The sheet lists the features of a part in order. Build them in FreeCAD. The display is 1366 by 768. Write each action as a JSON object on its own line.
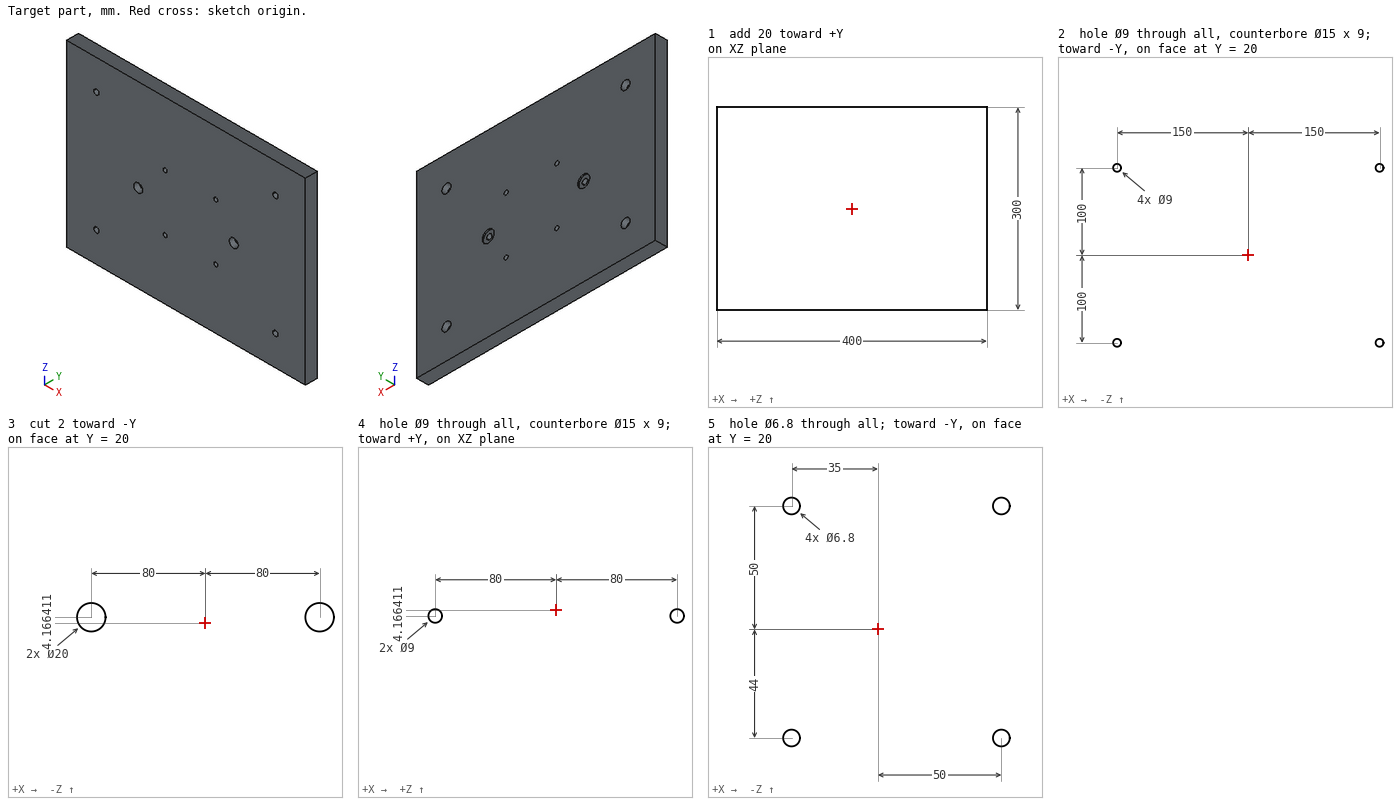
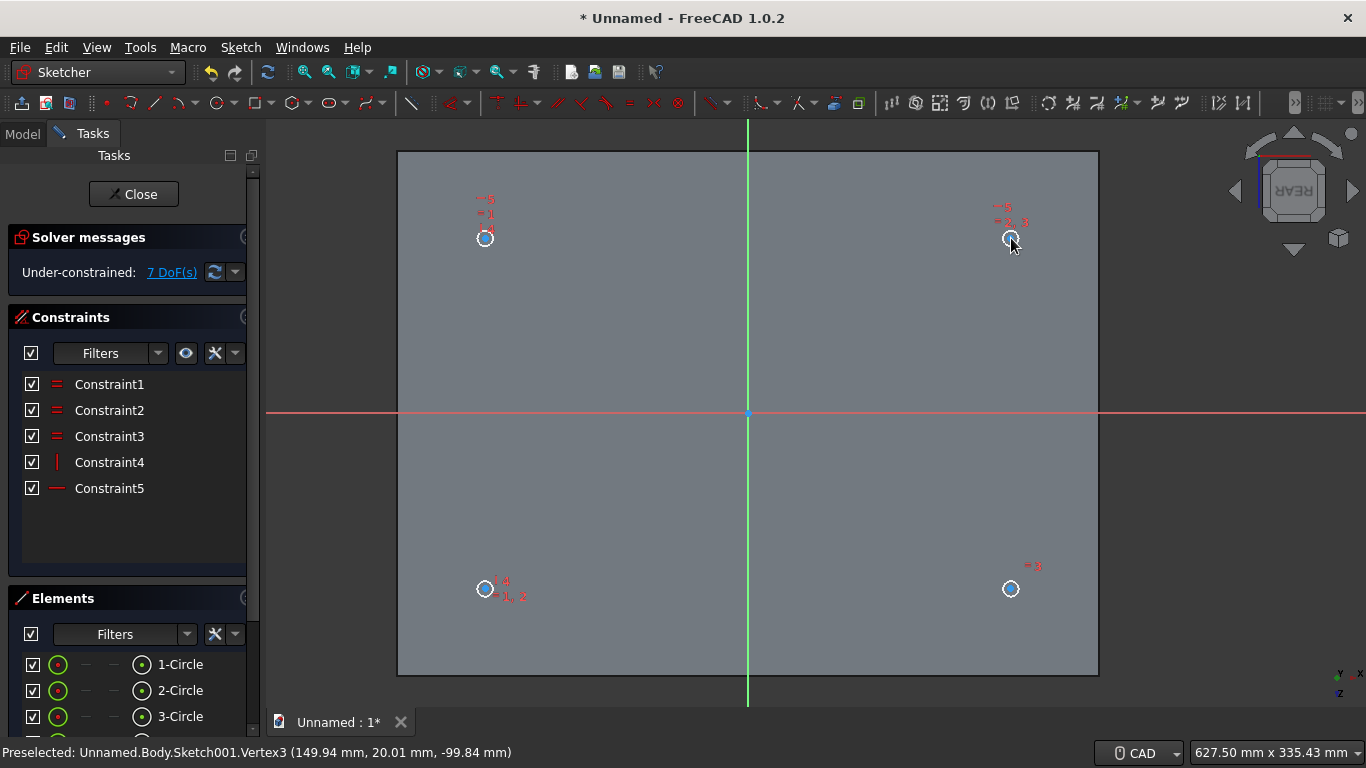
{"action": "left_click", "coordinate": [1011, 238]}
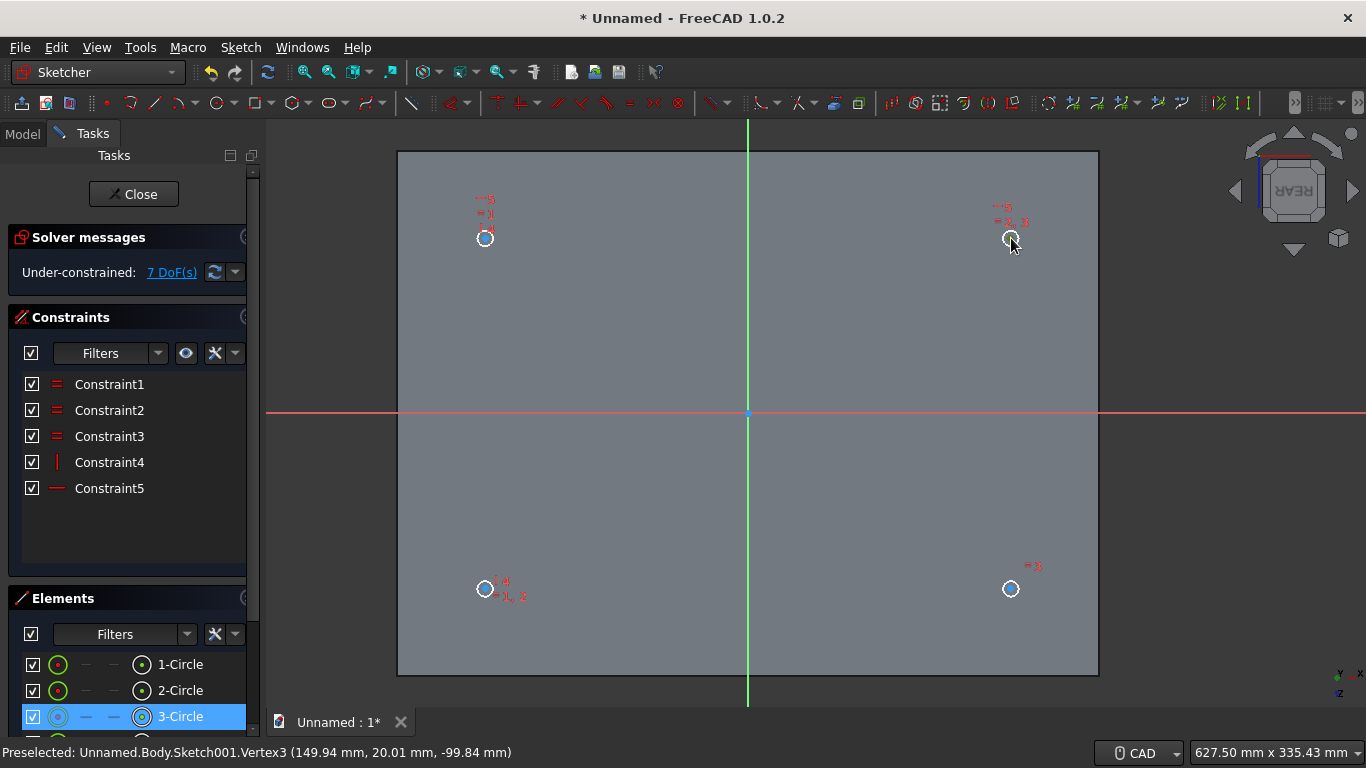
{"action": "left_click", "coordinate": [1011, 589]}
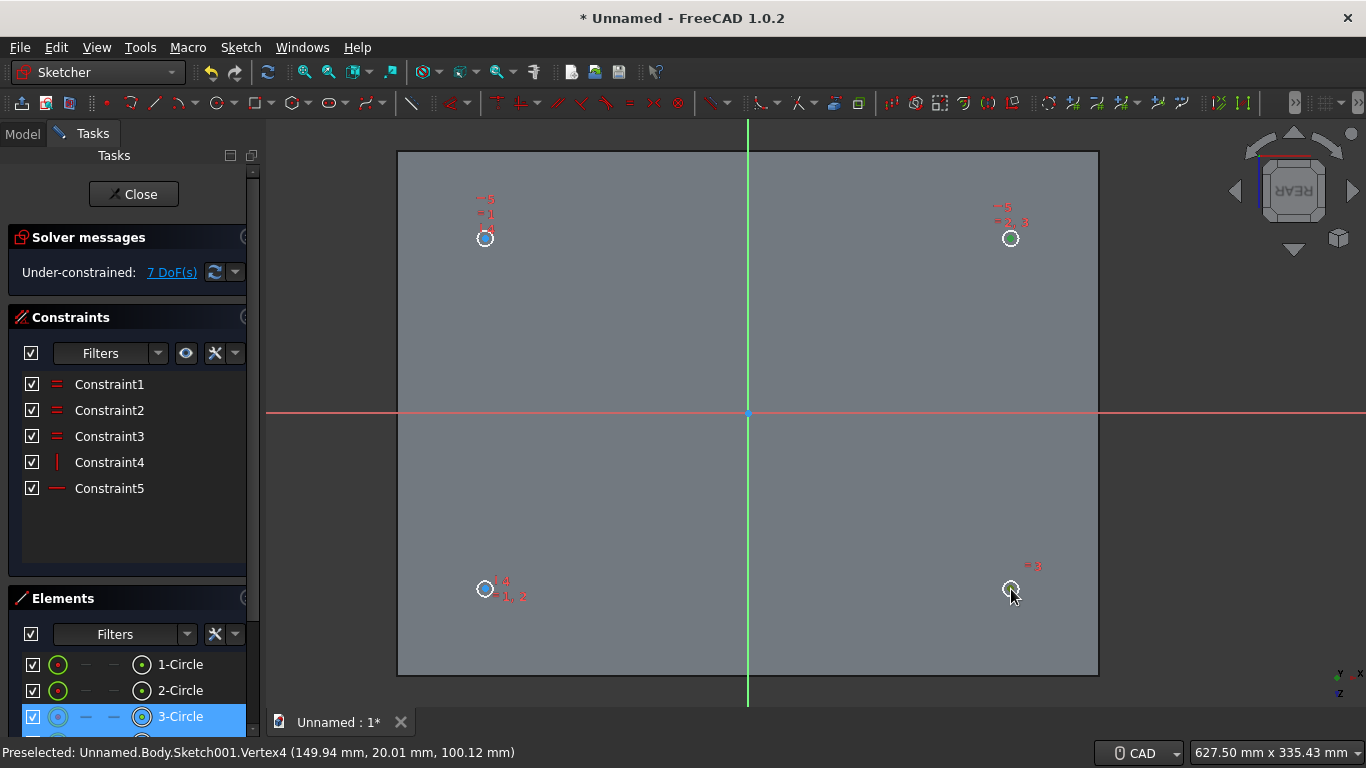
{"action": "key", "text": "v"}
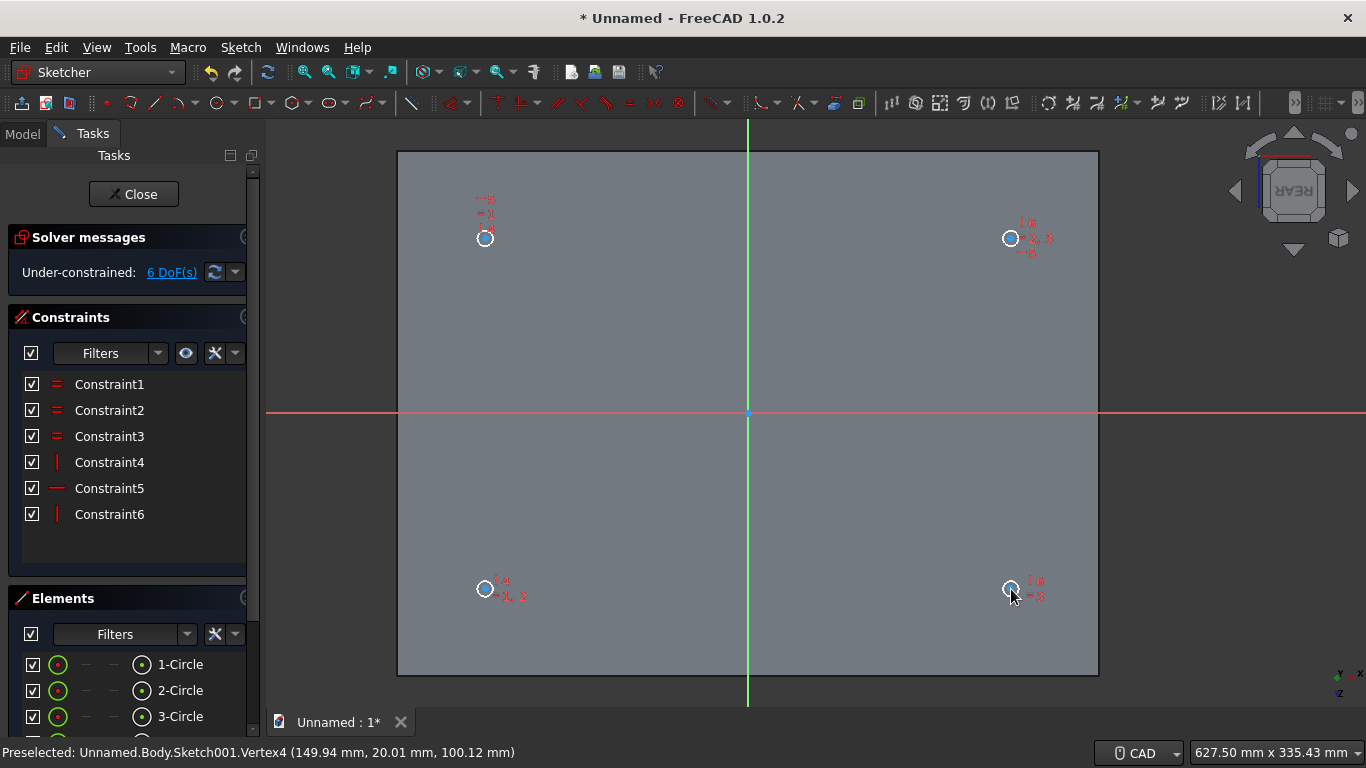
{"action": "left_click", "coordinate": [485, 589]}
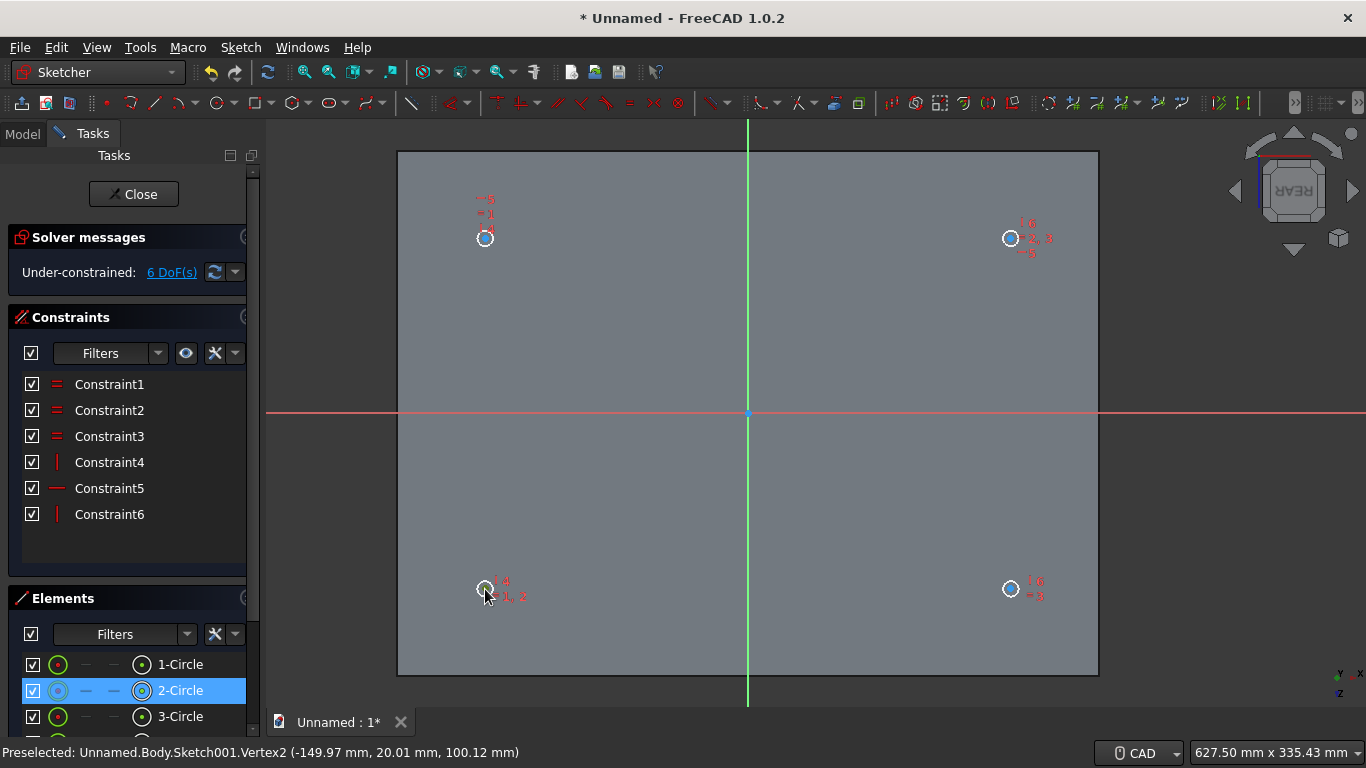
{"action": "left_click", "coordinate": [1011, 589]}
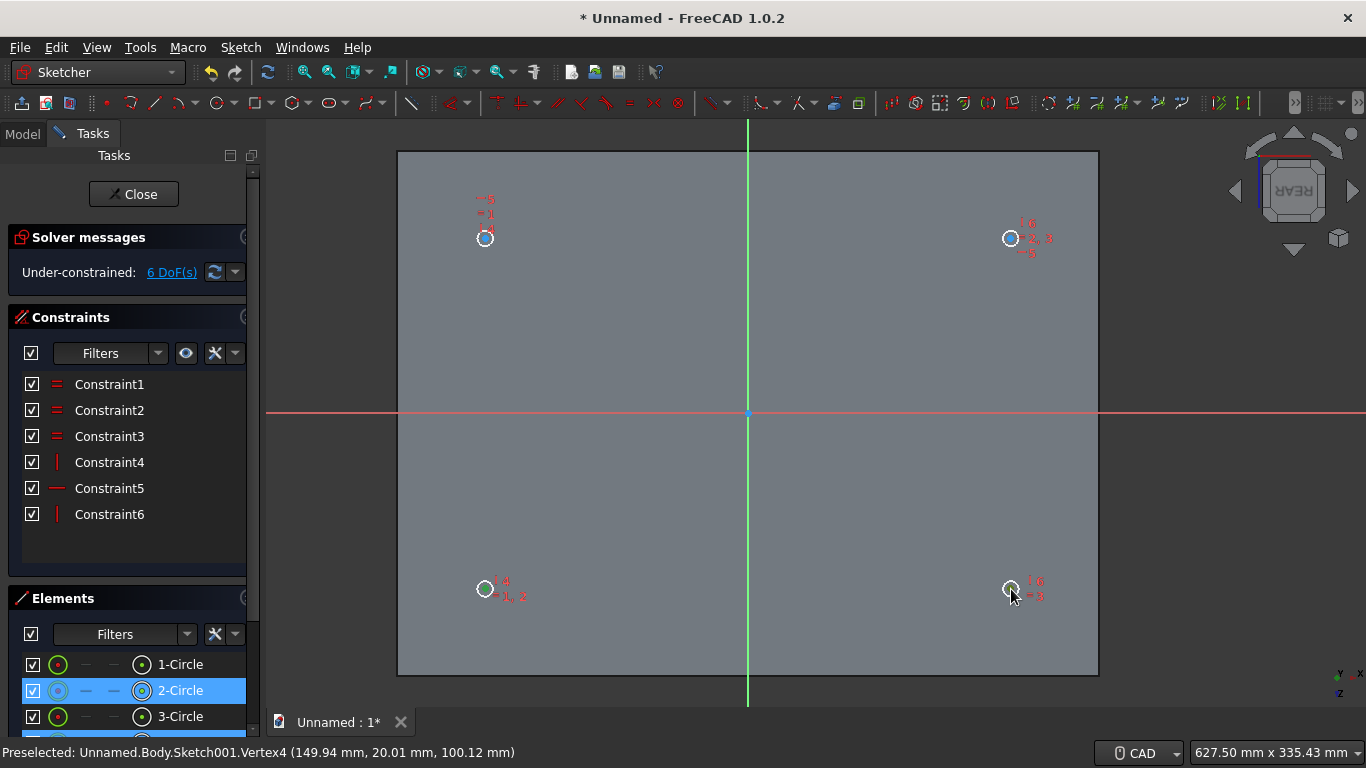
{"action": "left_click", "coordinate": [540, 104]}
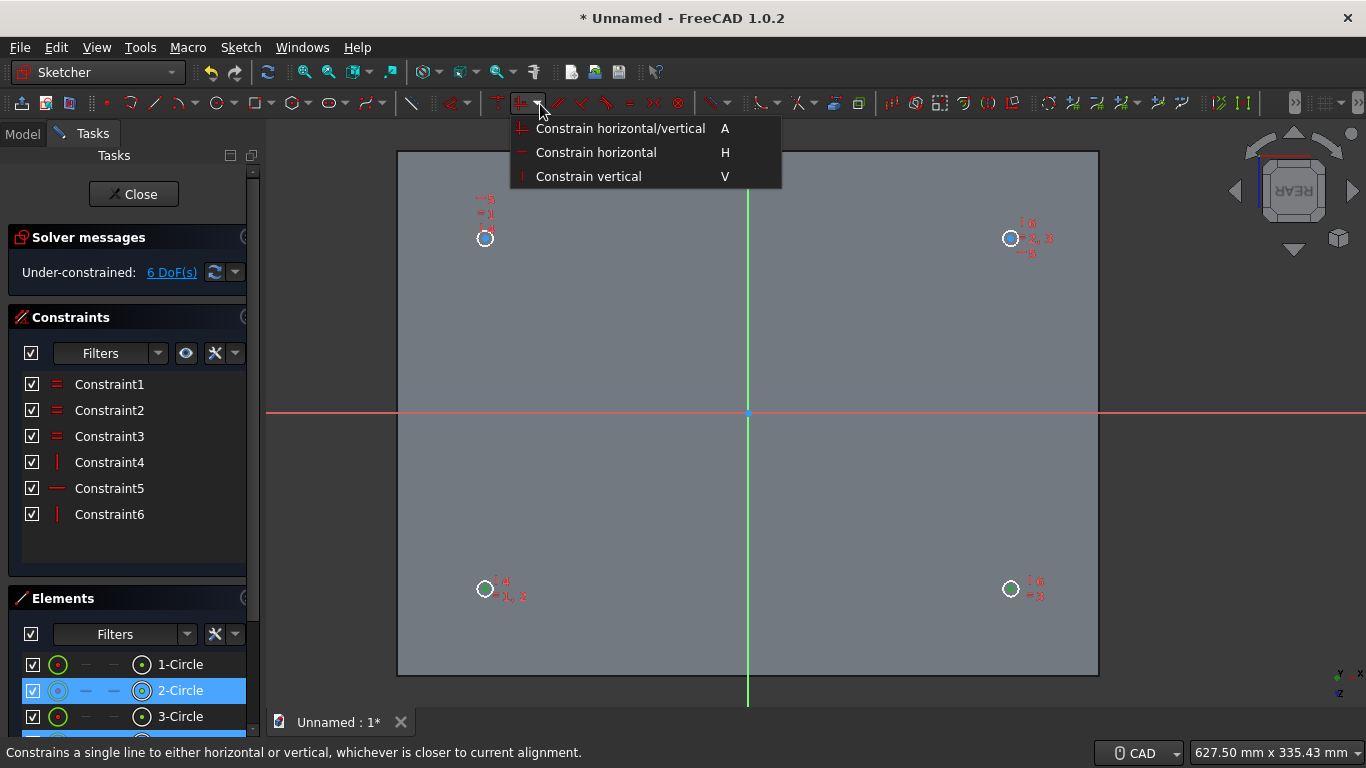
{"action": "left_click", "coordinate": [646, 152]}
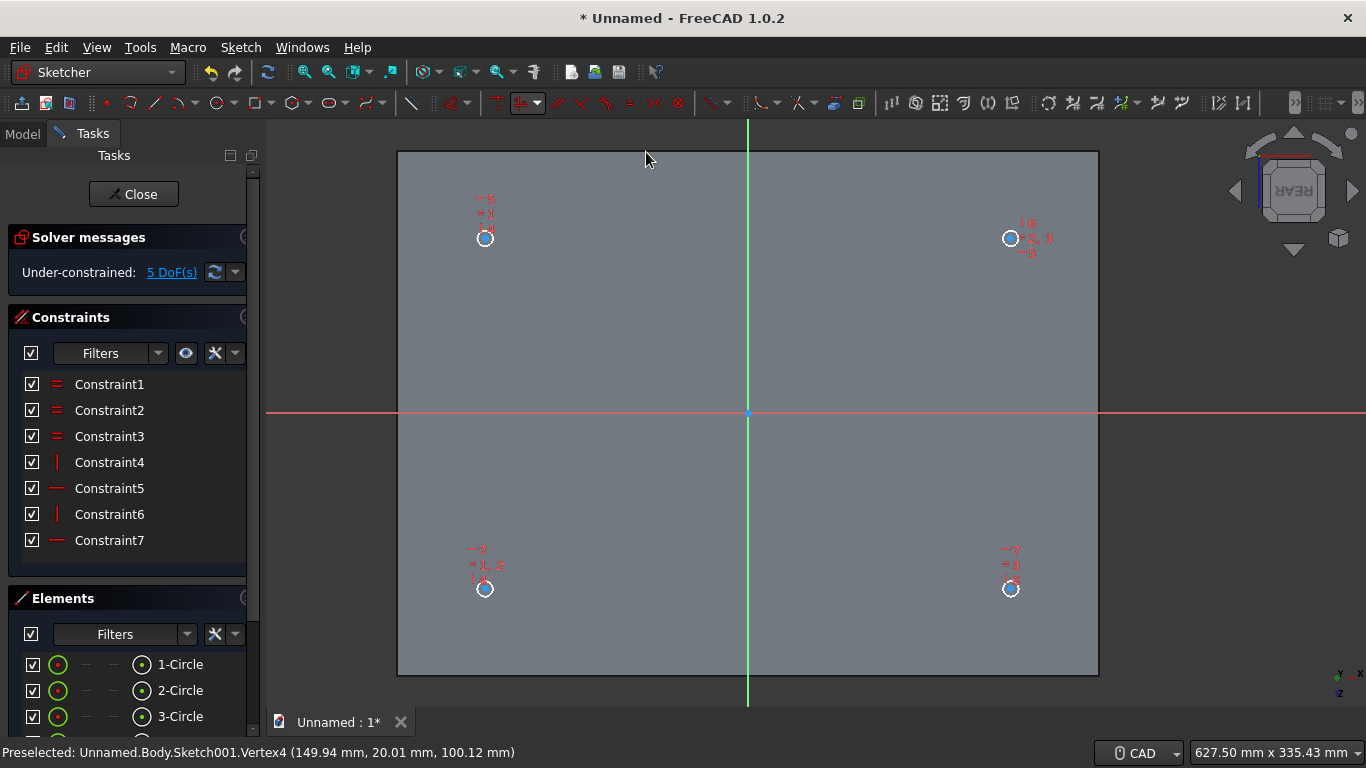
{"action": "left_click", "coordinate": [450, 104]}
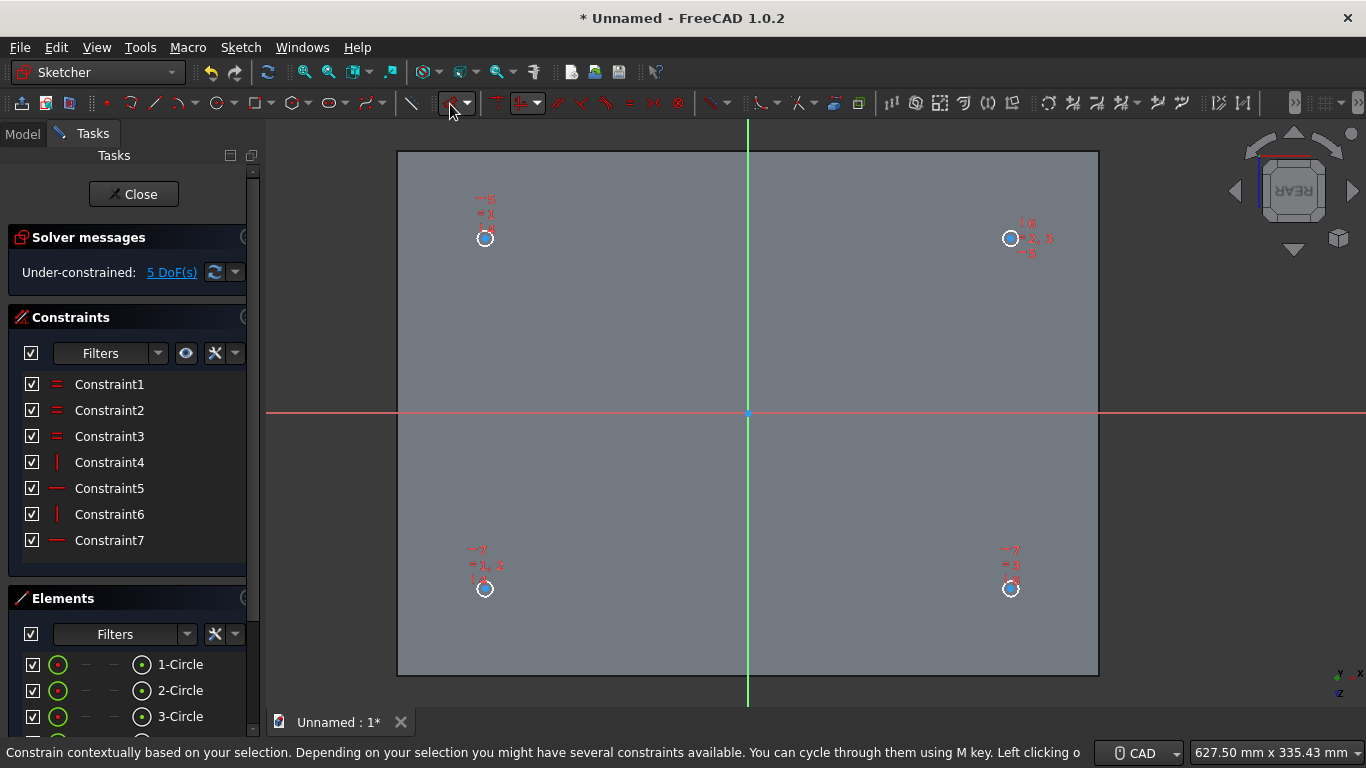
{"action": "scroll", "coordinate": [491, 233], "scroll_direction": "up", "scroll_amount": 5}